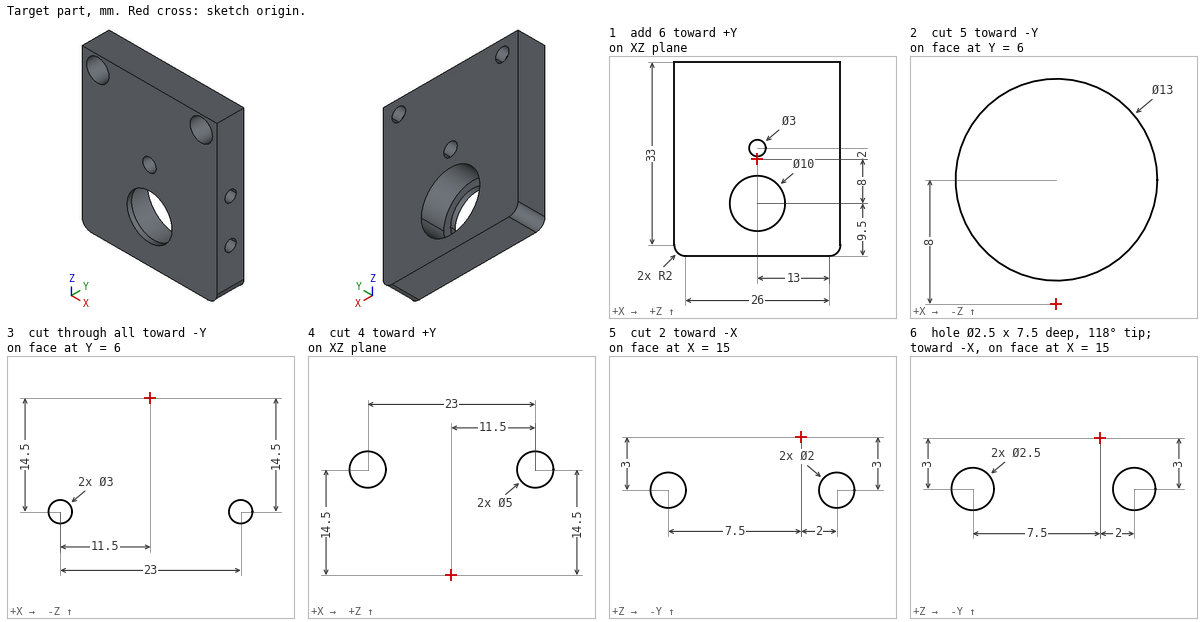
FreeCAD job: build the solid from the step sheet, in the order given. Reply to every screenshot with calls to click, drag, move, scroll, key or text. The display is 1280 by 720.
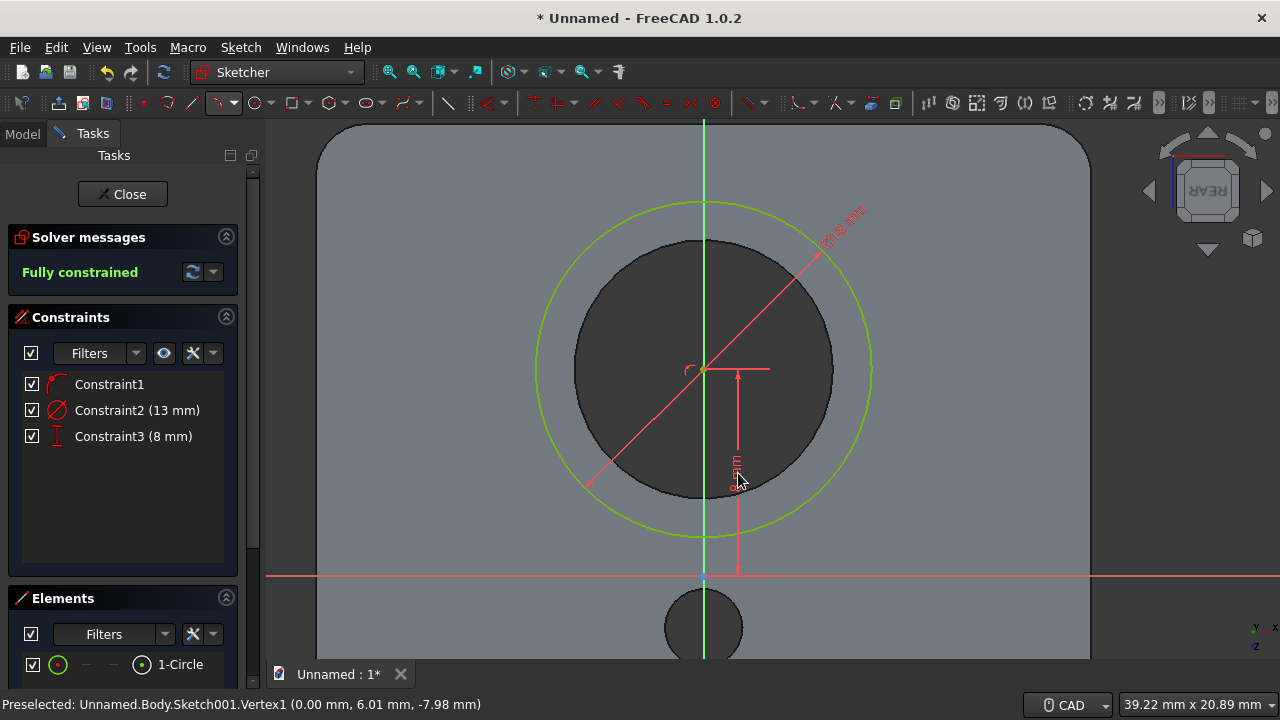
click(123, 194)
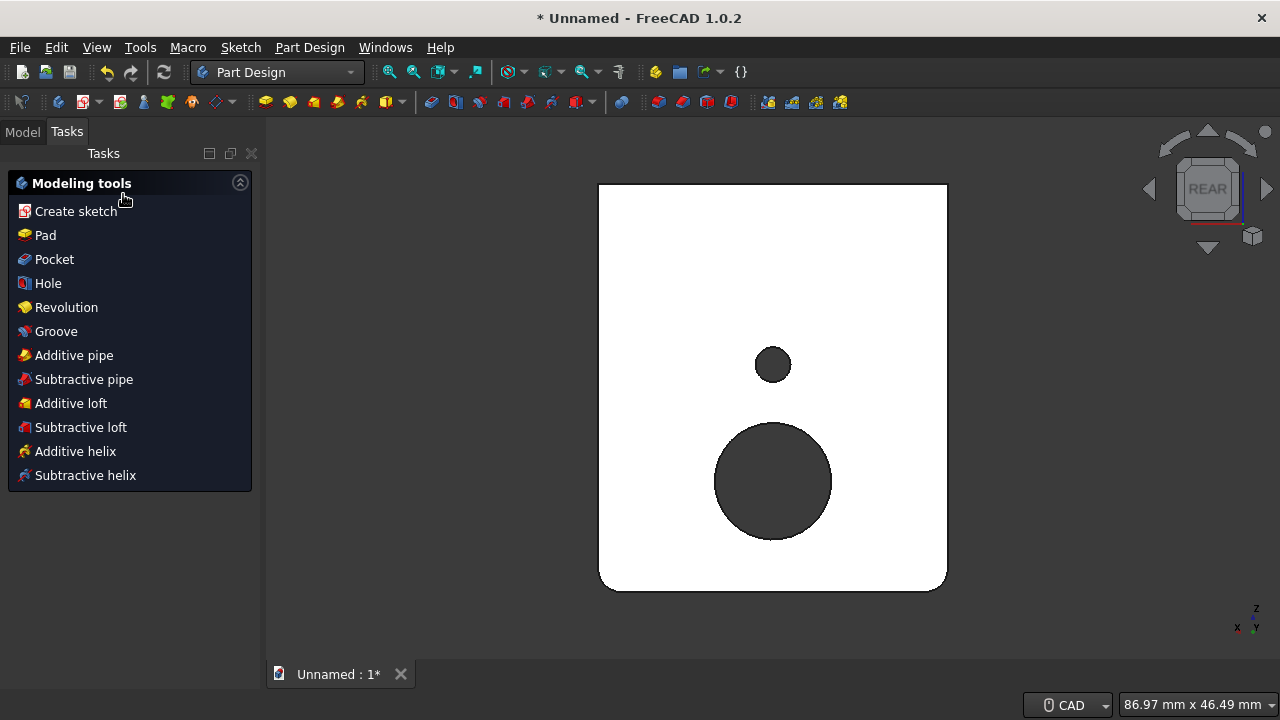
click(432, 102)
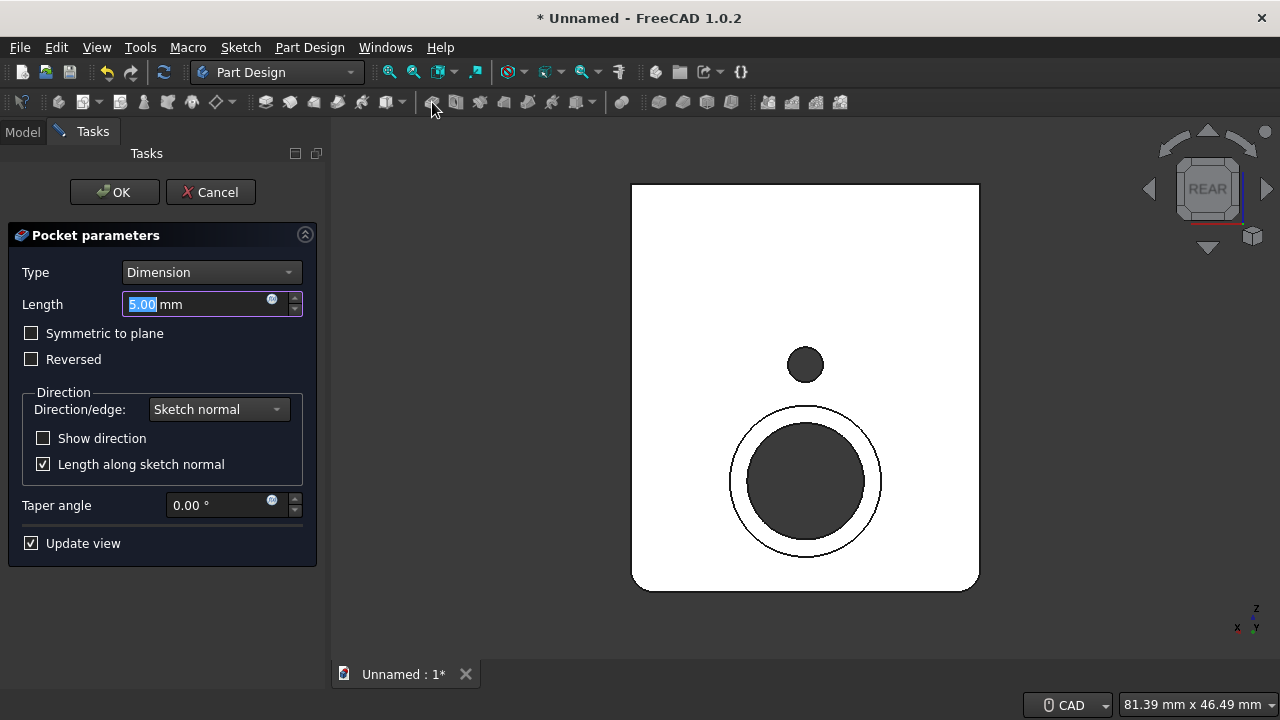
text(5)
key(Tab)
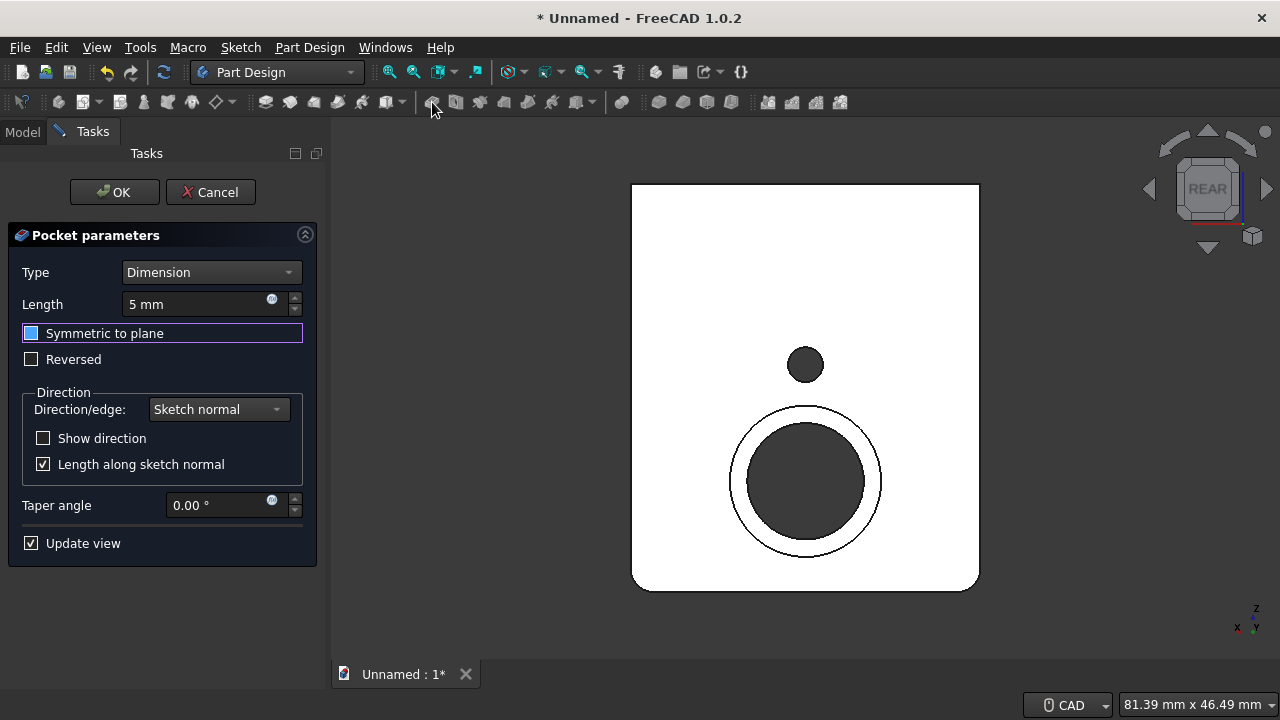
click(115, 192)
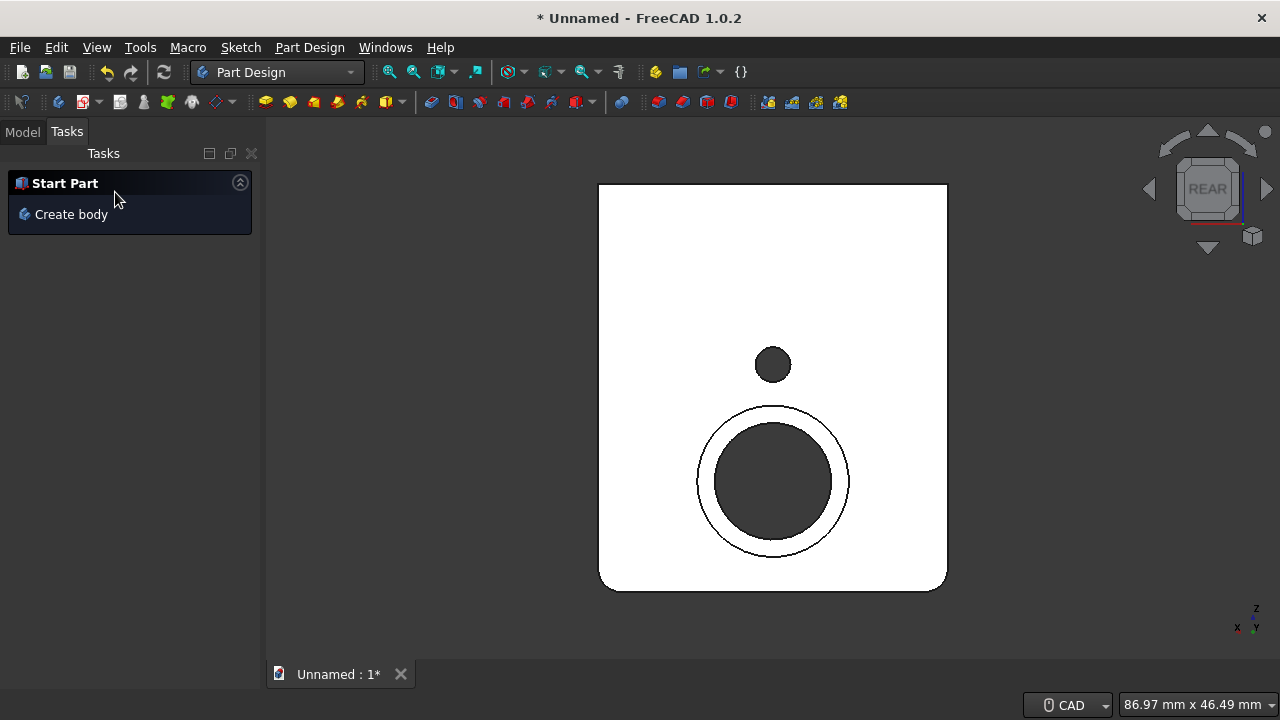
click(723, 270)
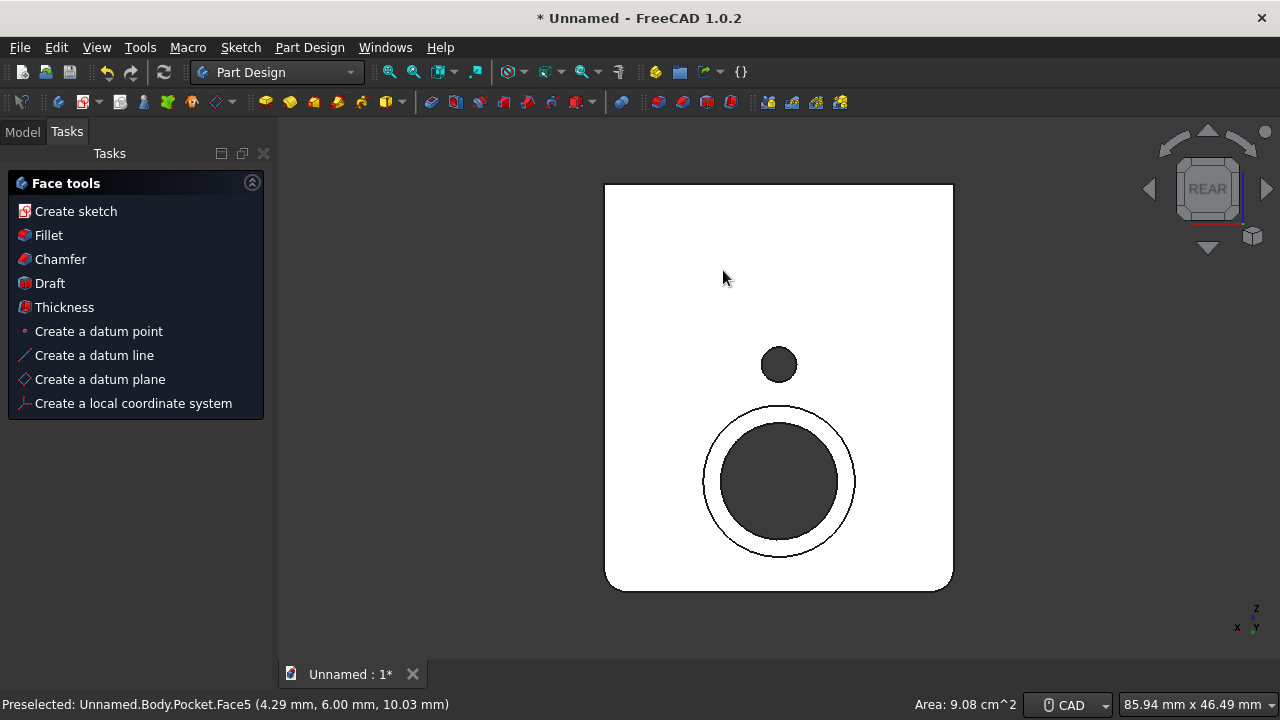
click(84, 102)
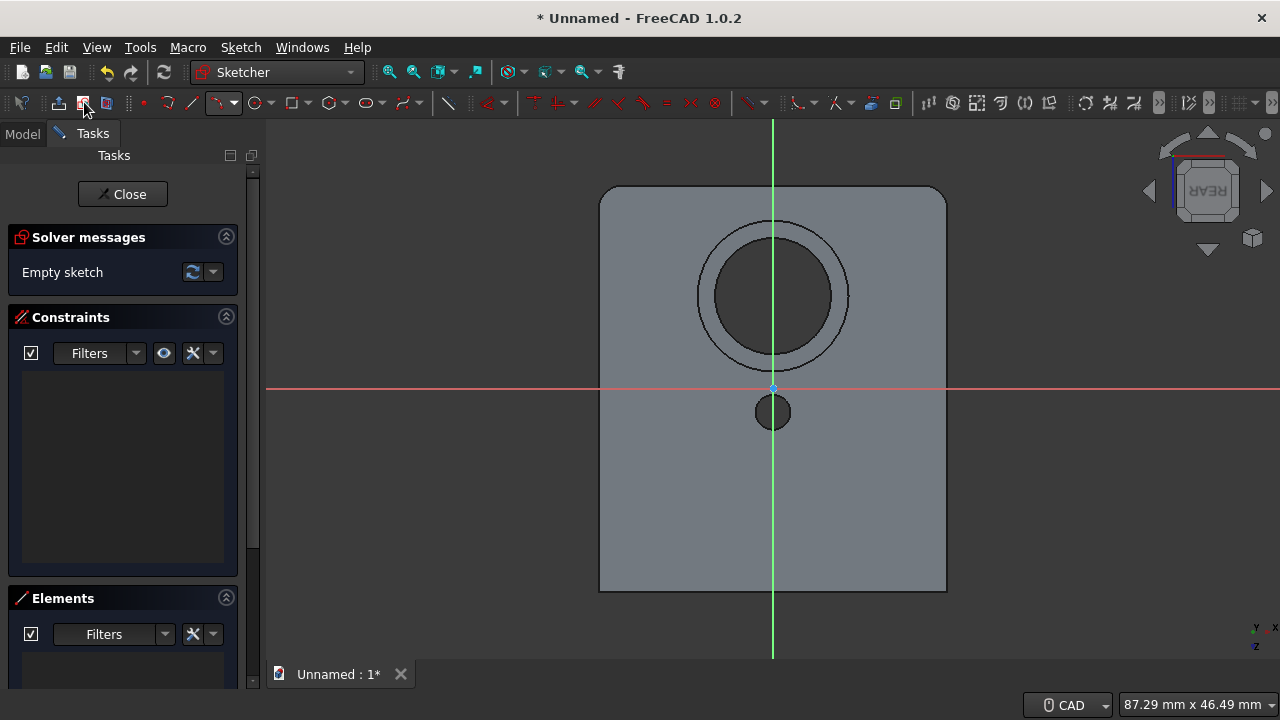
scroll(856, 595, up, 3)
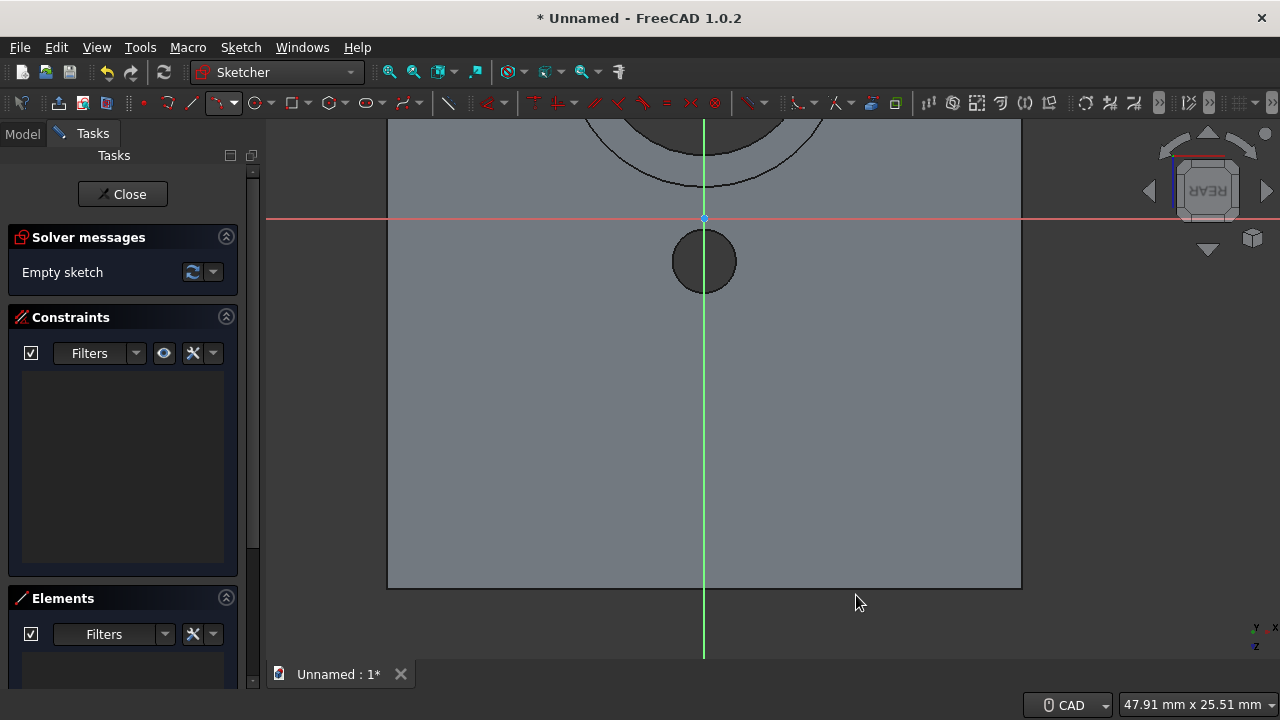
click(256, 104)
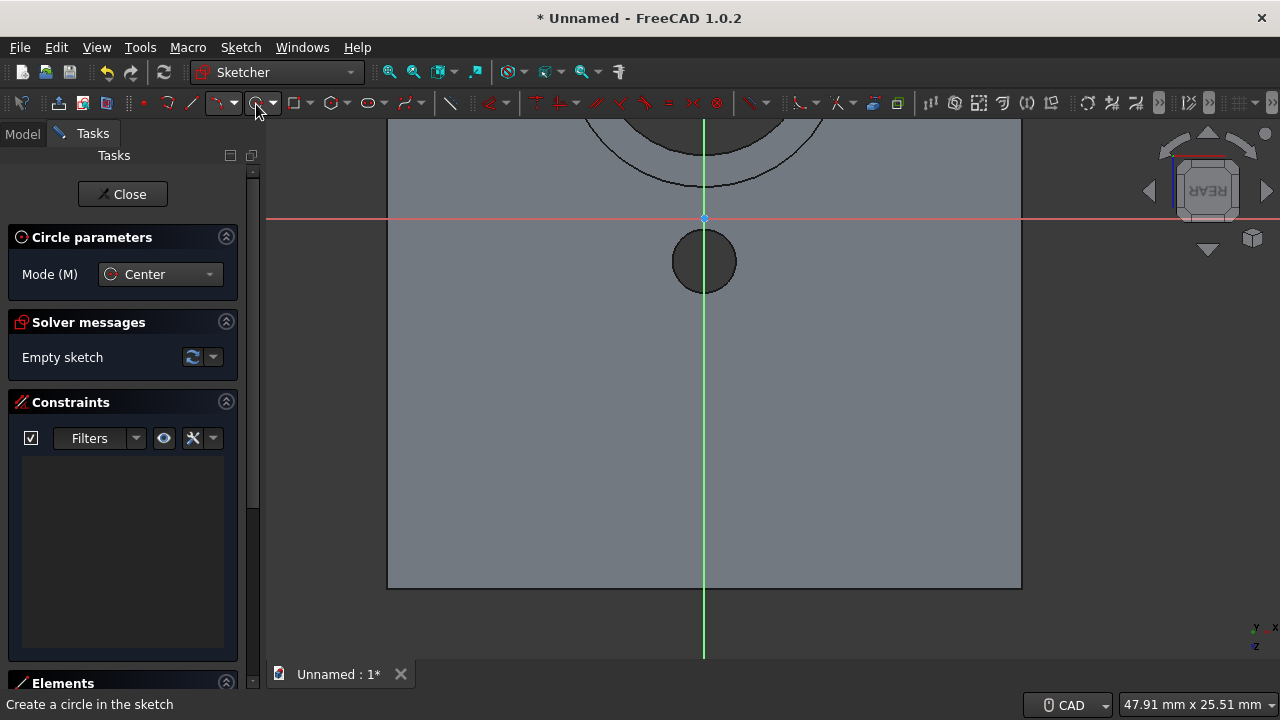
click(461, 526)
click(483, 503)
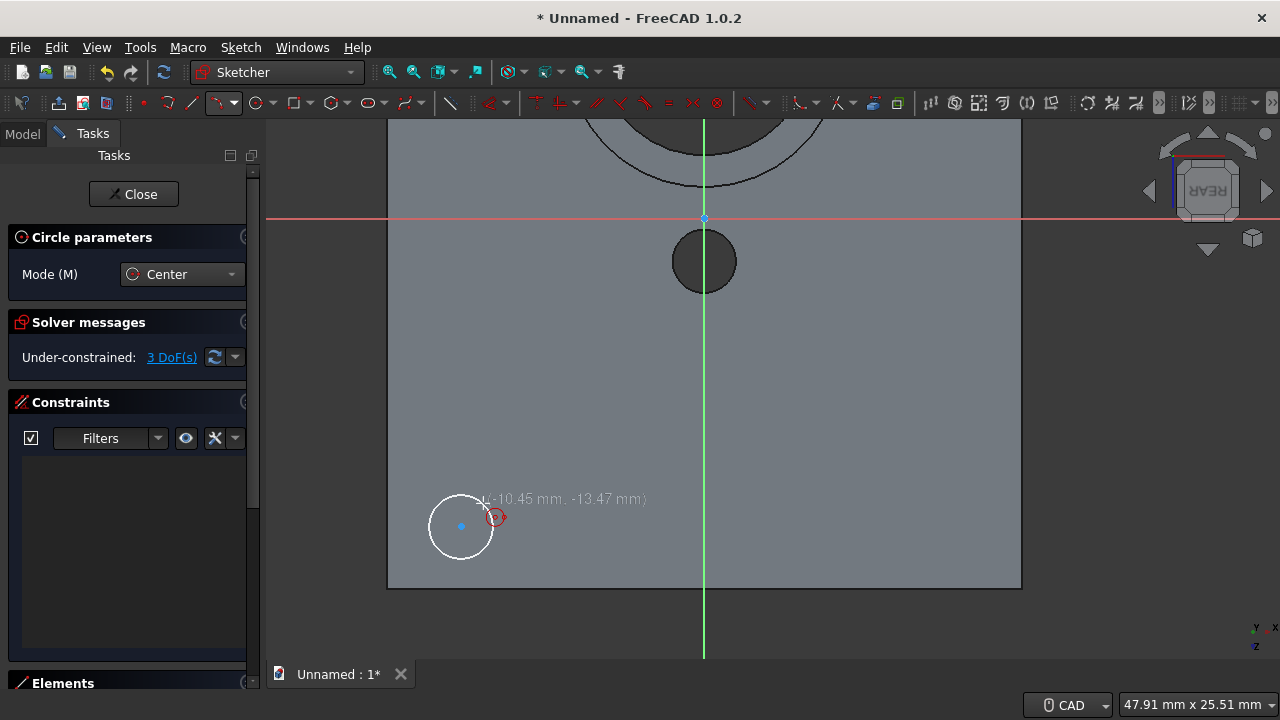
click(948, 526)
click(970, 503)
key(Escape)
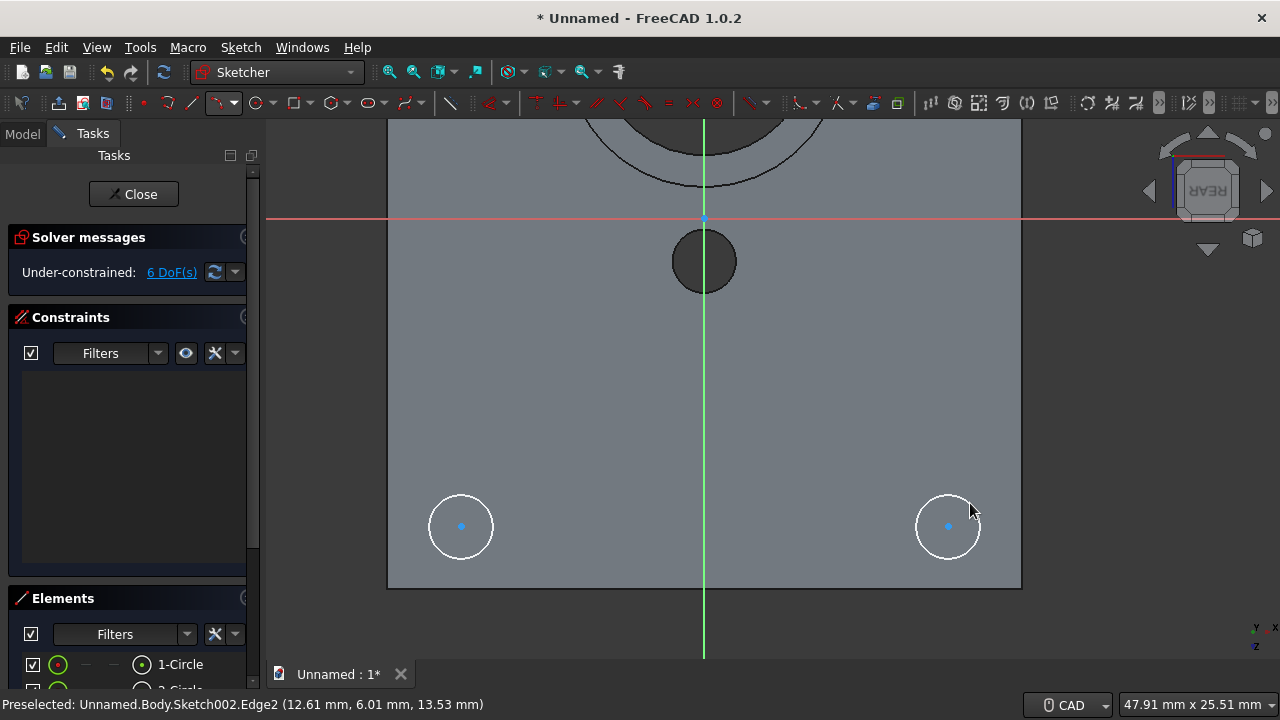
click(483, 504)